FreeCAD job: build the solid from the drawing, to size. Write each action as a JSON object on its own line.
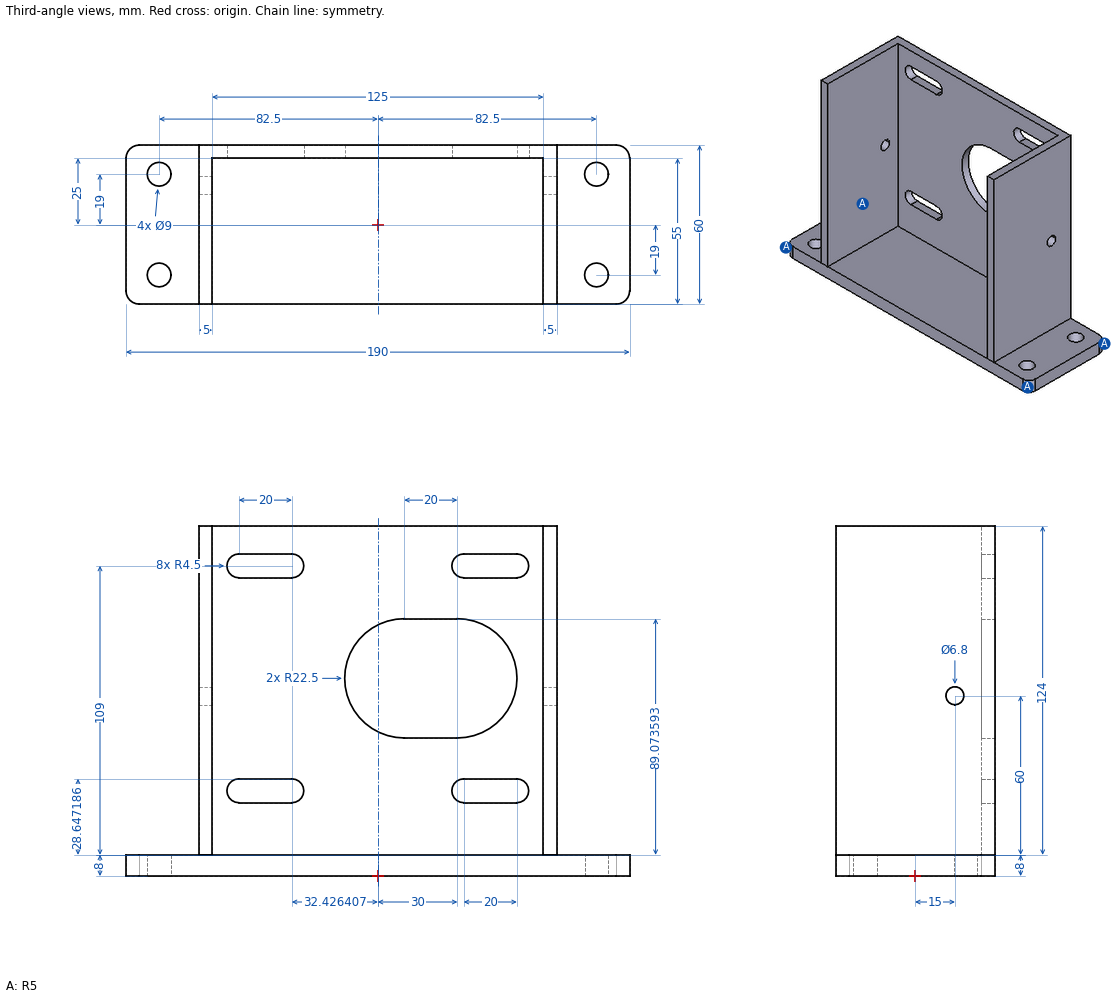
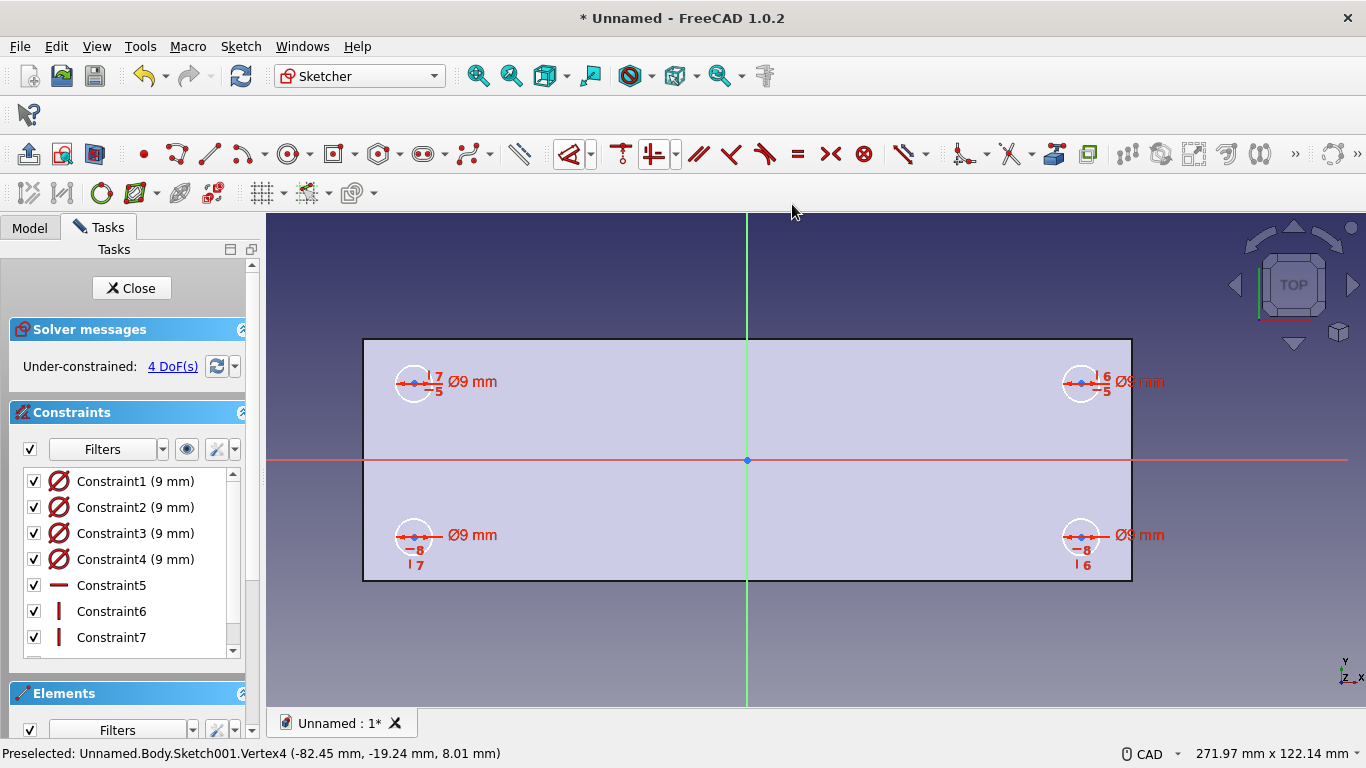
{"action": "key", "text": "d"}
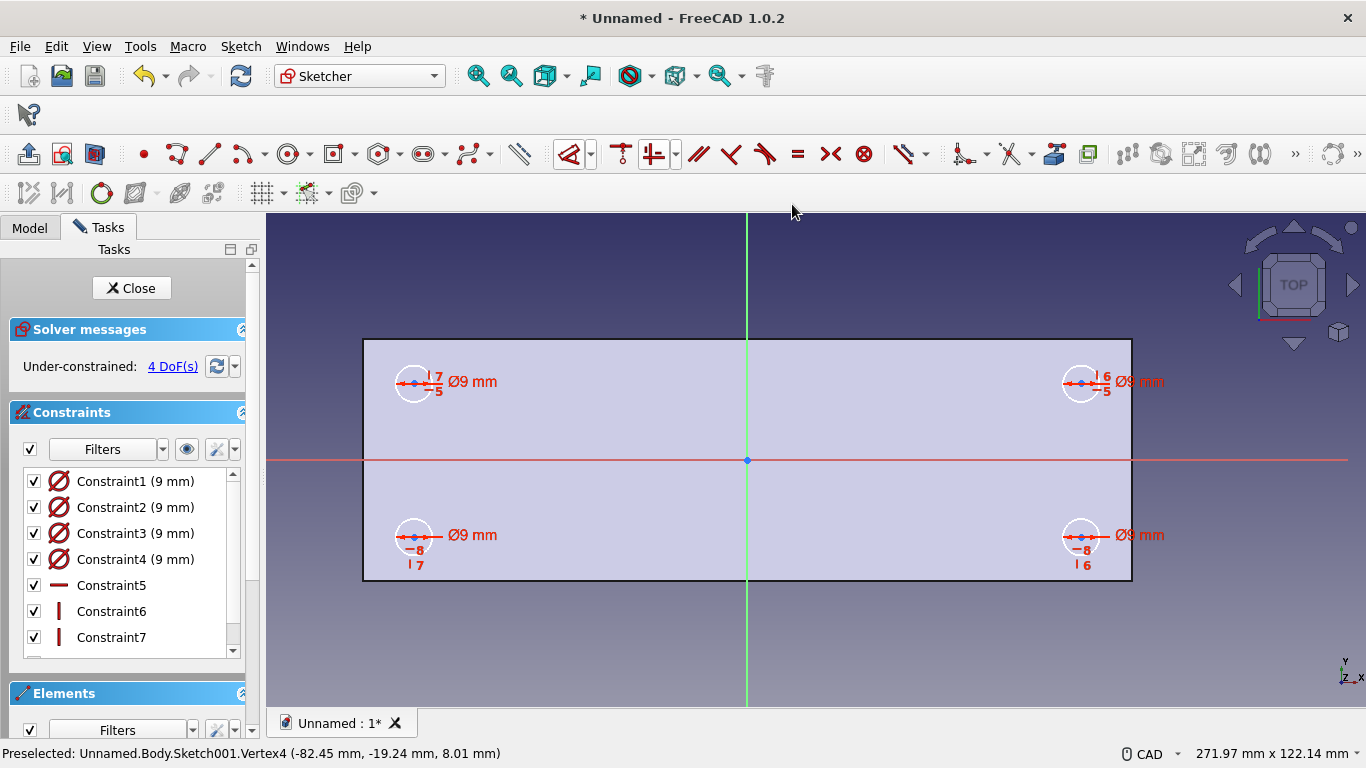
{"action": "left_click", "coordinate": [414, 384]}
{"action": "left_click", "coordinate": [380, 422]}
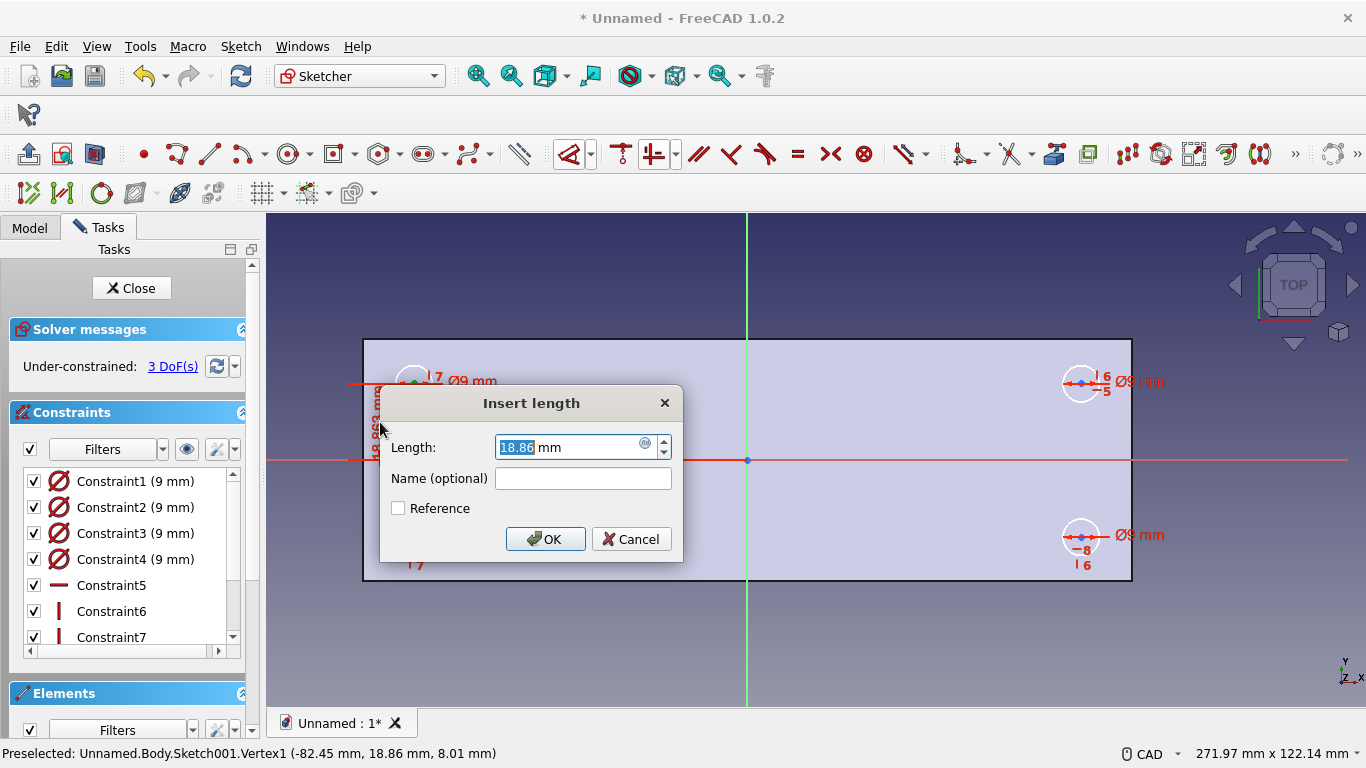
{"action": "type", "text": "19"}
{"action": "key", "text": "Return"}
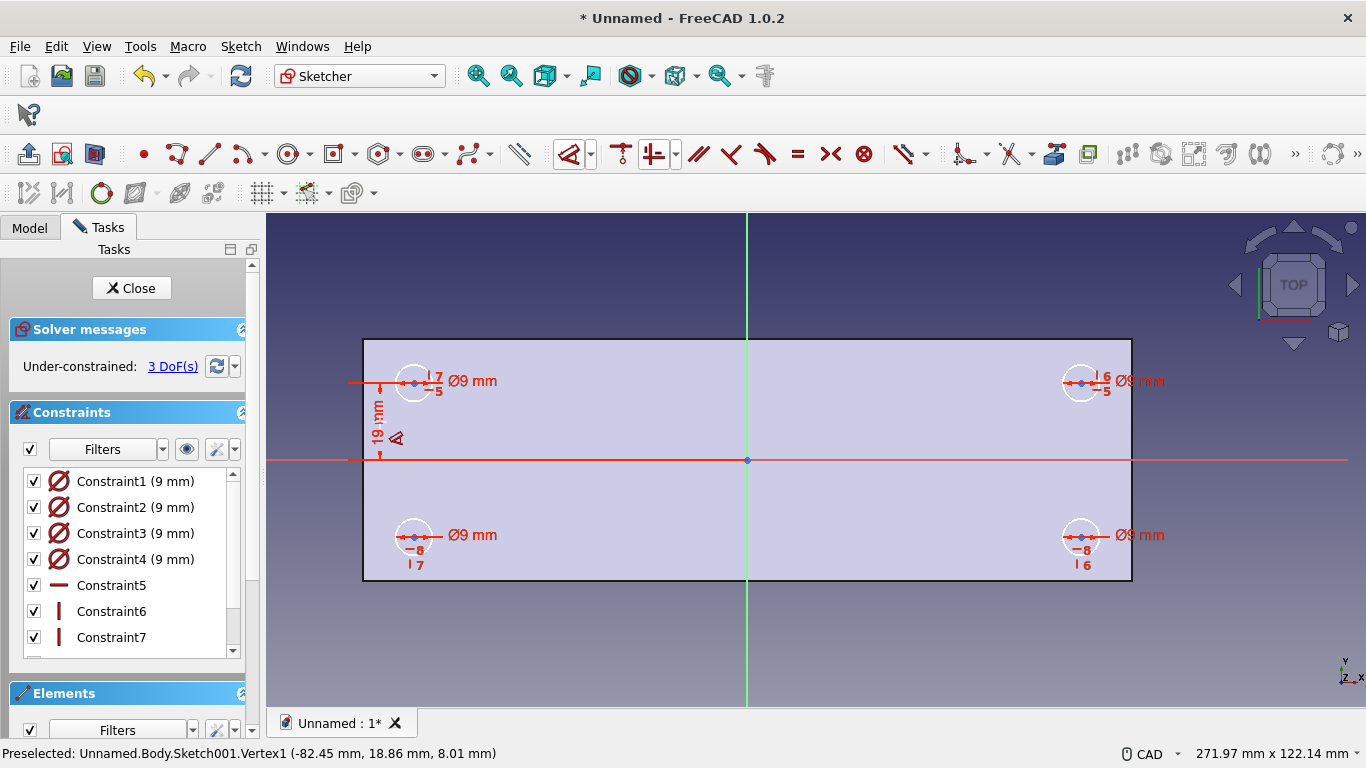
{"action": "left_click", "coordinate": [1081, 537]}
{"action": "left_click", "coordinate": [1115, 499]}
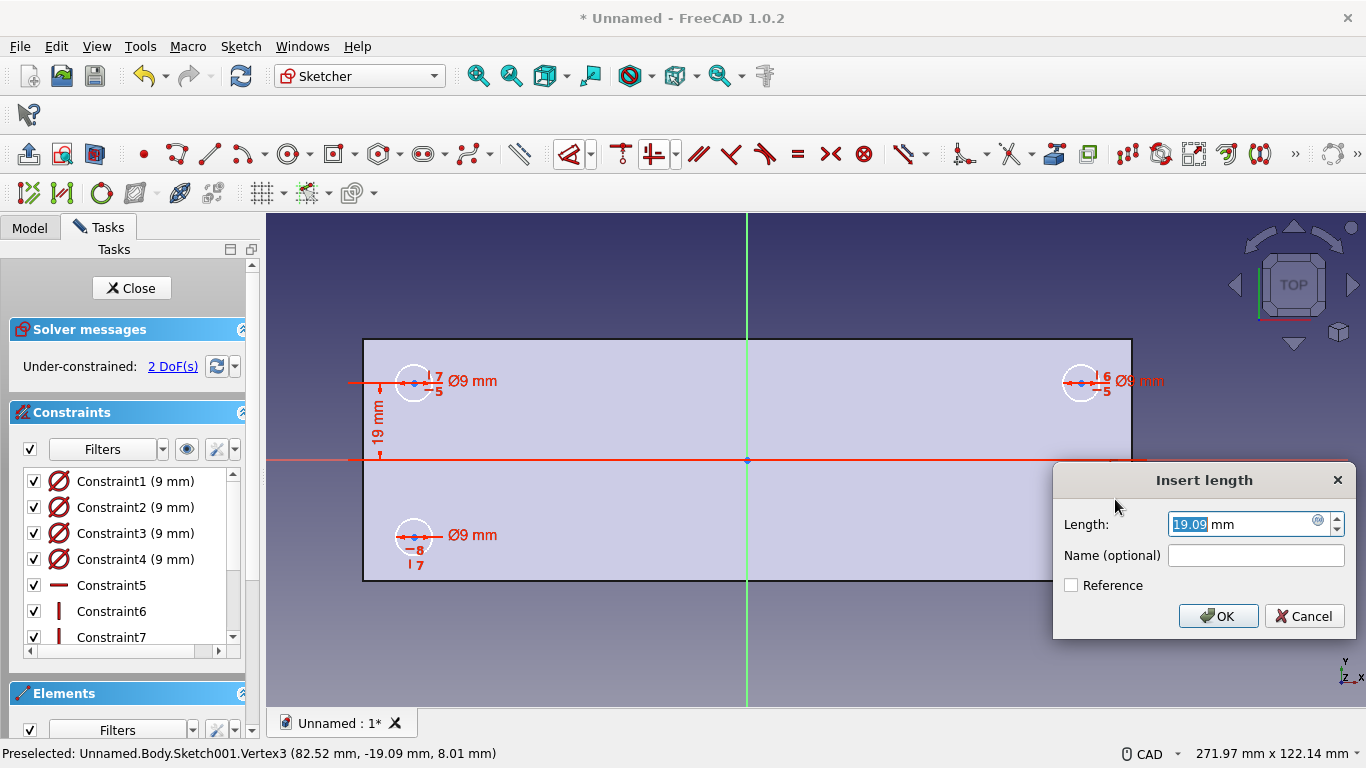
{"action": "type", "text": "19"}
{"action": "key", "text": "Return"}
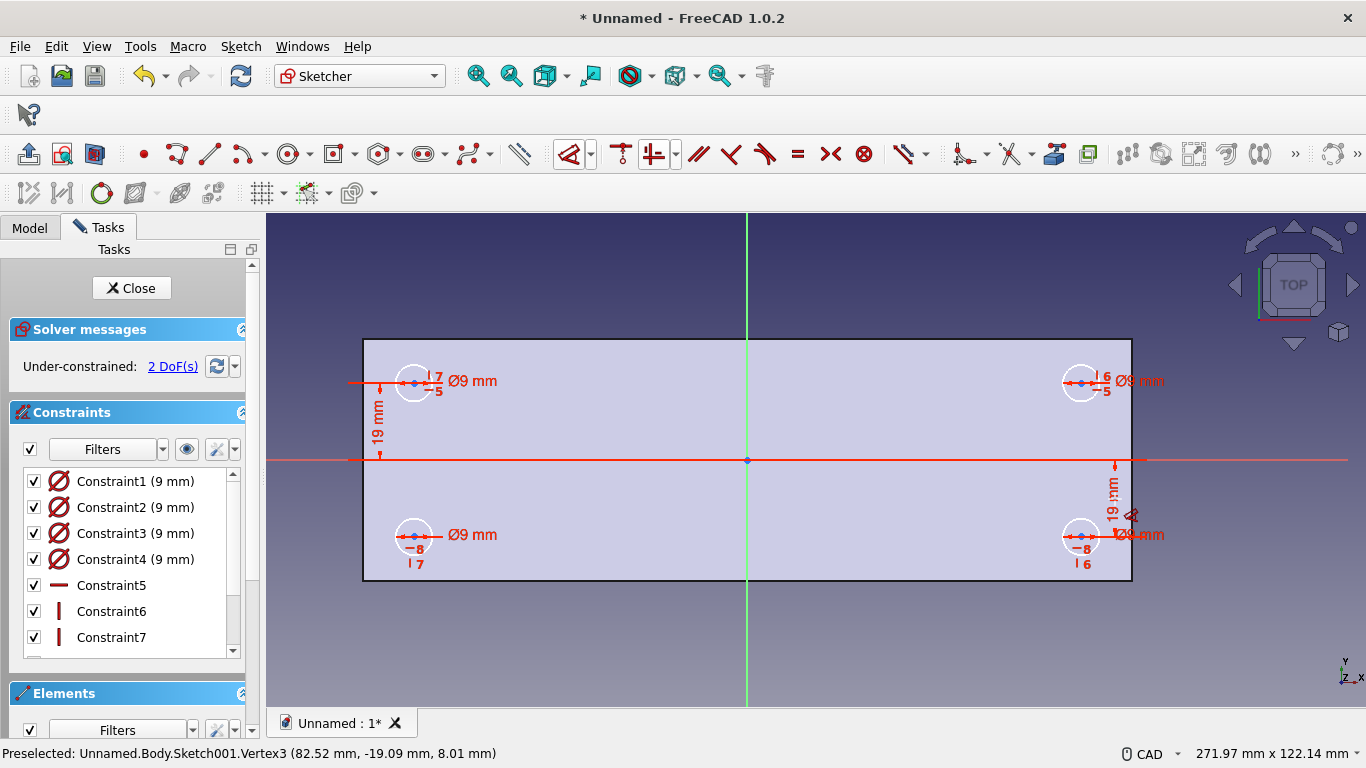
{"action": "left_click", "coordinate": [414, 383]}
{"action": "left_click", "coordinate": [581, 349]}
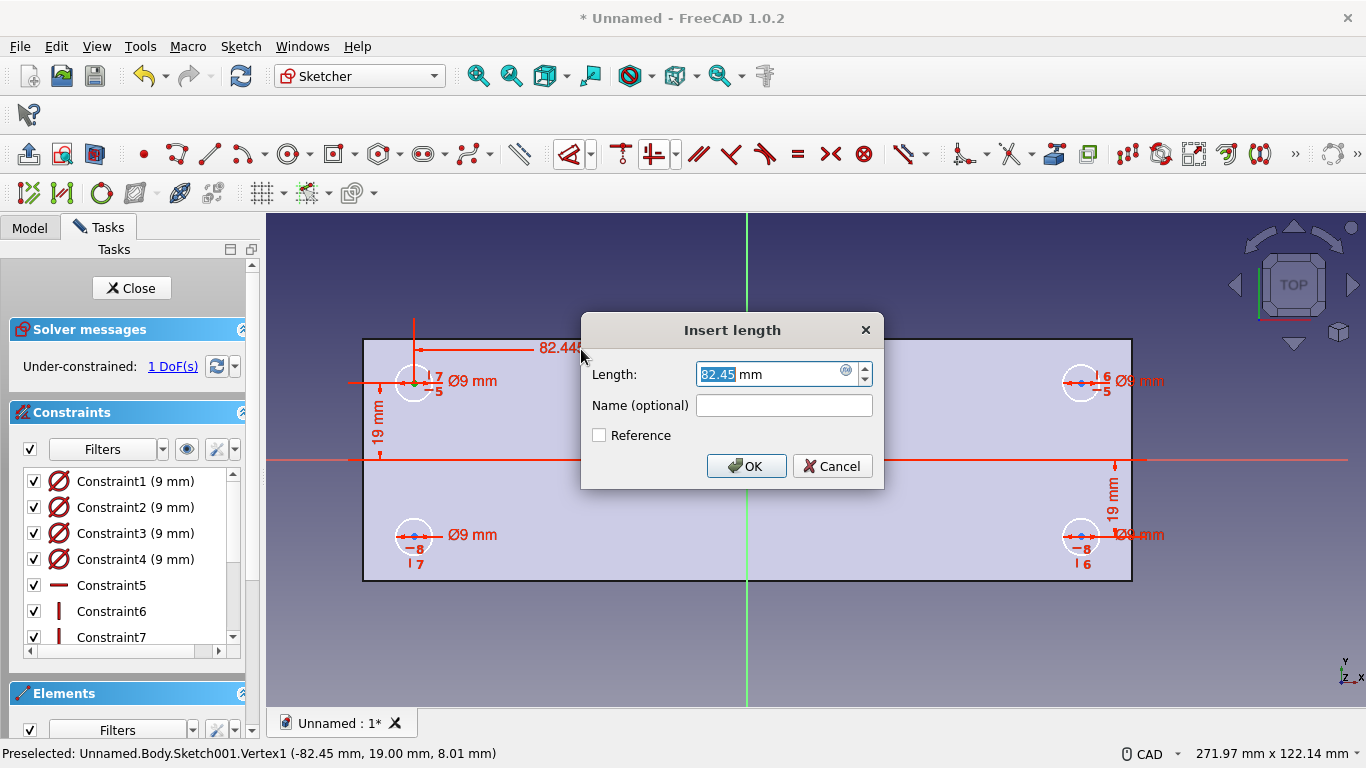
{"action": "type", "text": "82.5"}
{"action": "key", "text": "Return"}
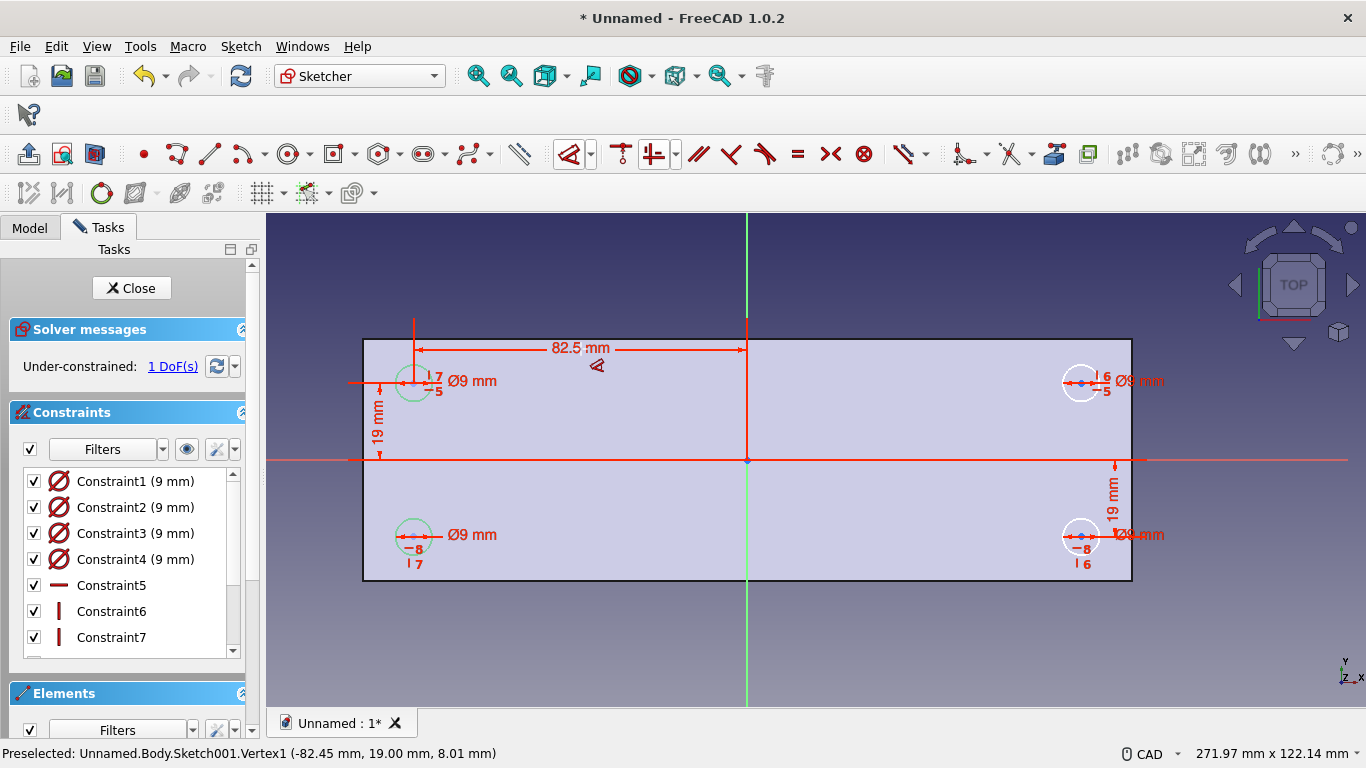
{"action": "left_click", "coordinate": [1081, 383]}
{"action": "left_click", "coordinate": [914, 349]}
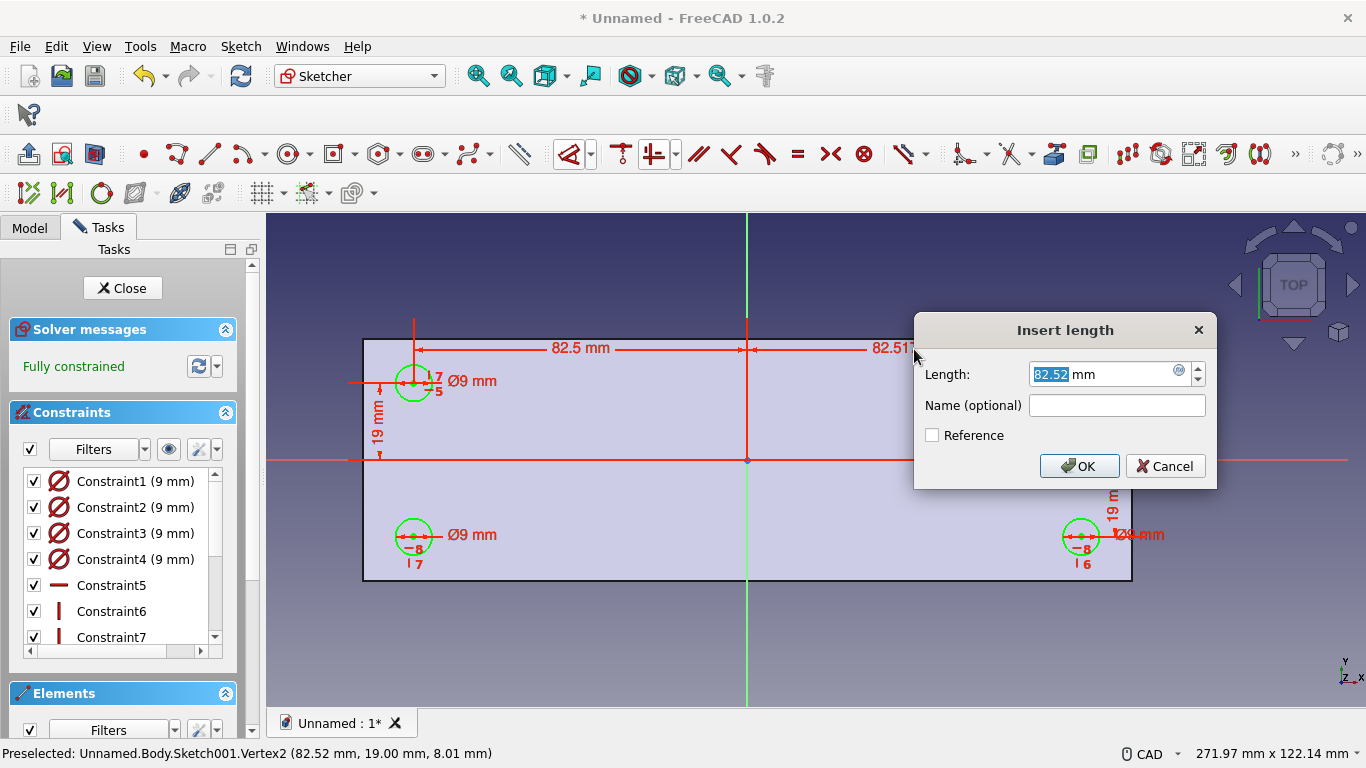
{"action": "type", "text": "82.5"}
{"action": "key", "text": "Return"}
{"action": "key", "text": "Escape"}